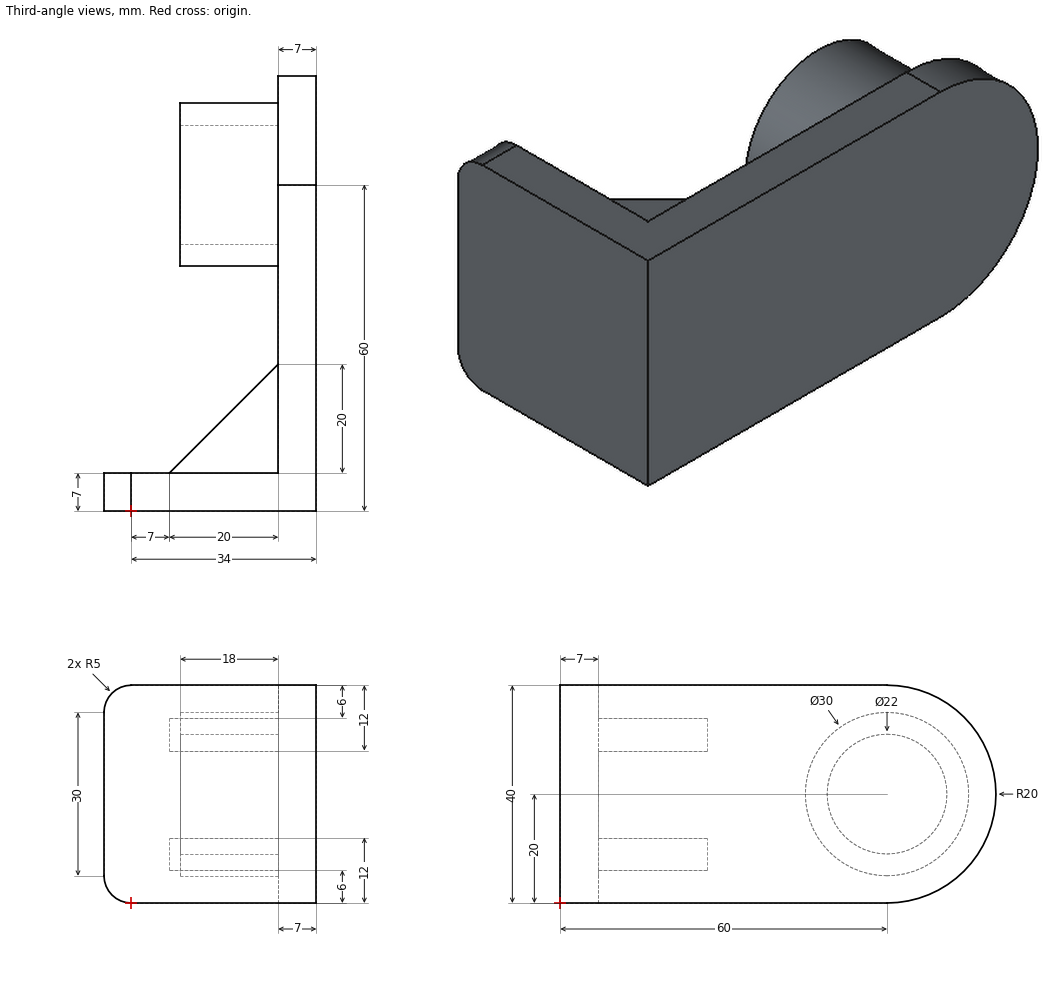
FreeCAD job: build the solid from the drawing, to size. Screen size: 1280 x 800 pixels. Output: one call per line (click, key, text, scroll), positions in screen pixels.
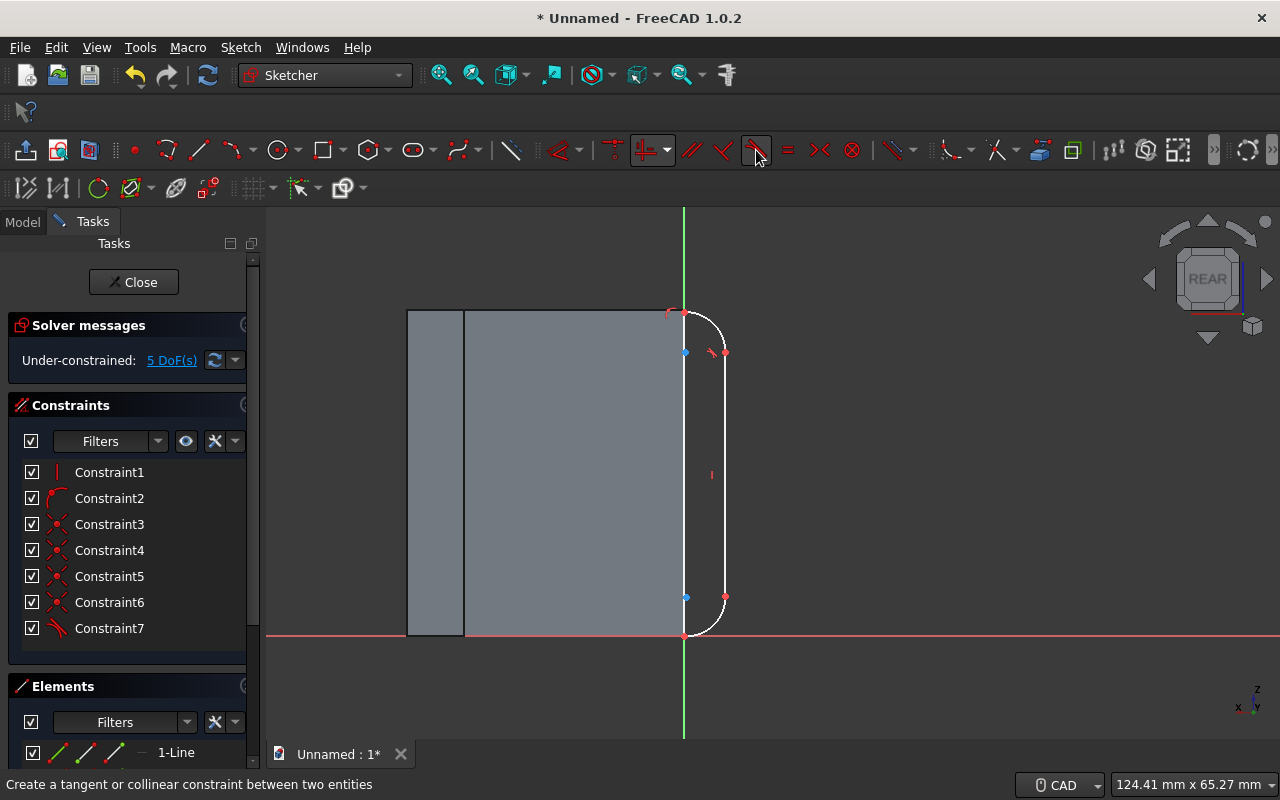
click(725, 523)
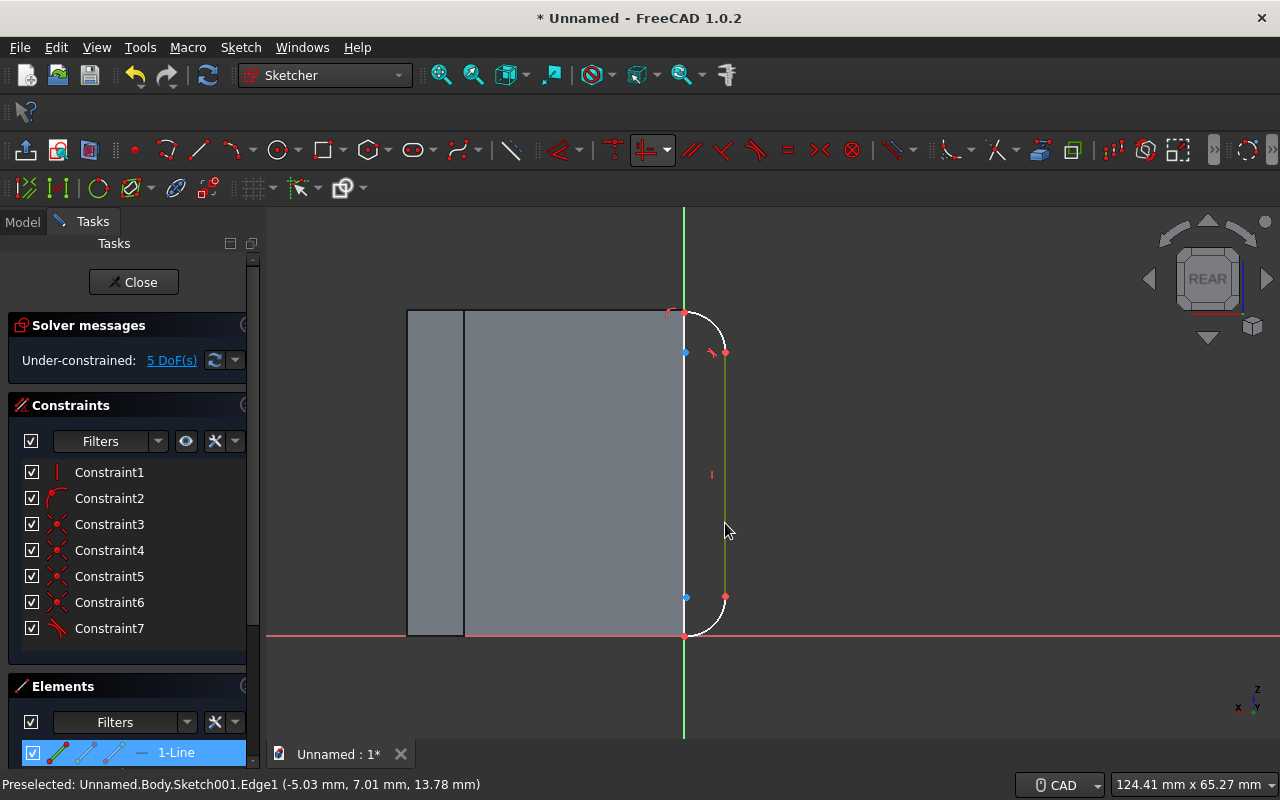
click(703, 633)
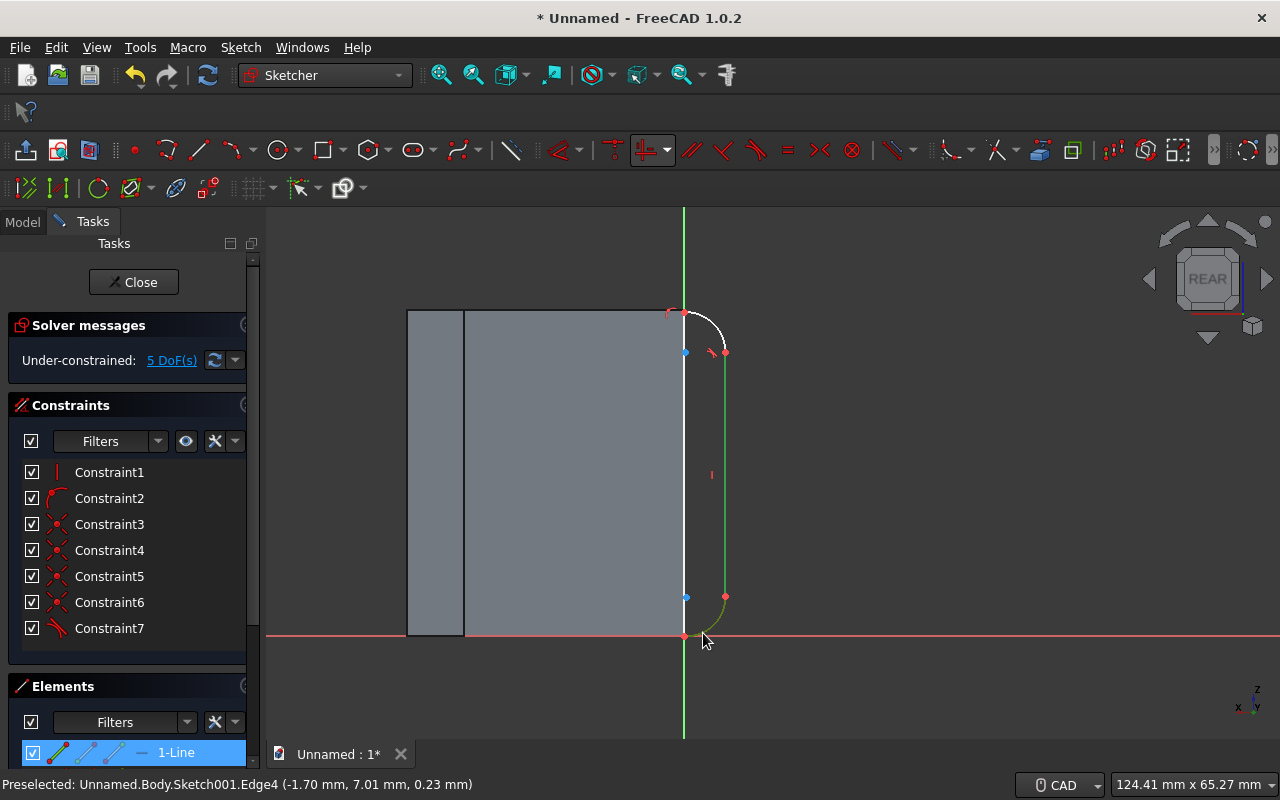
click(756, 150)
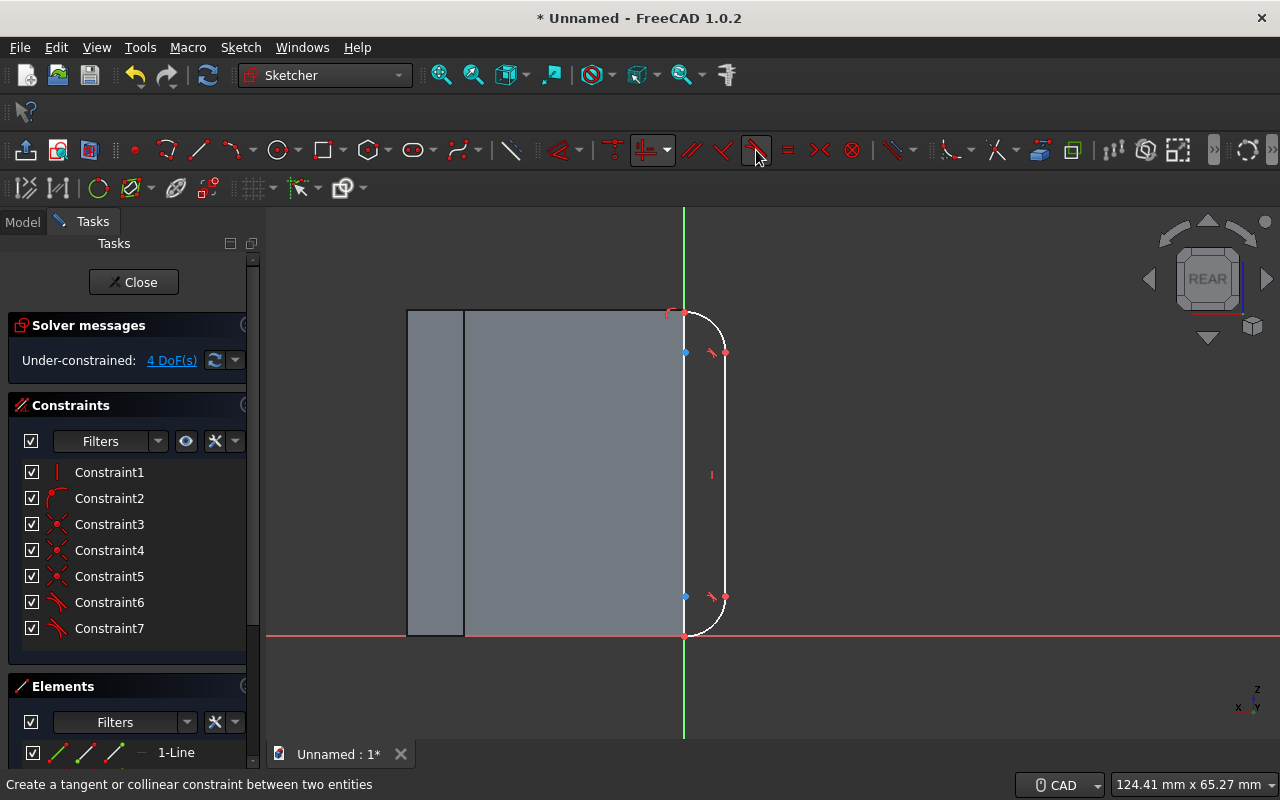
click(721, 334)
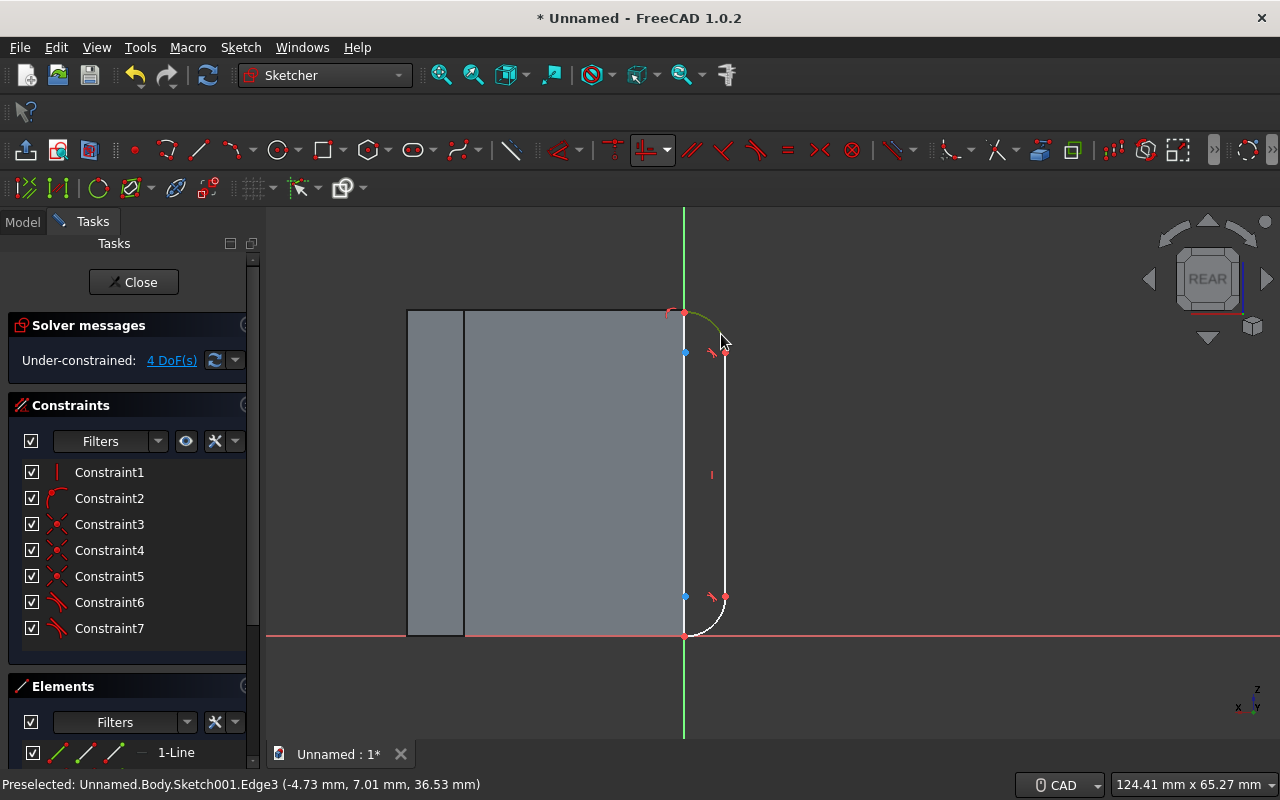
click(703, 632)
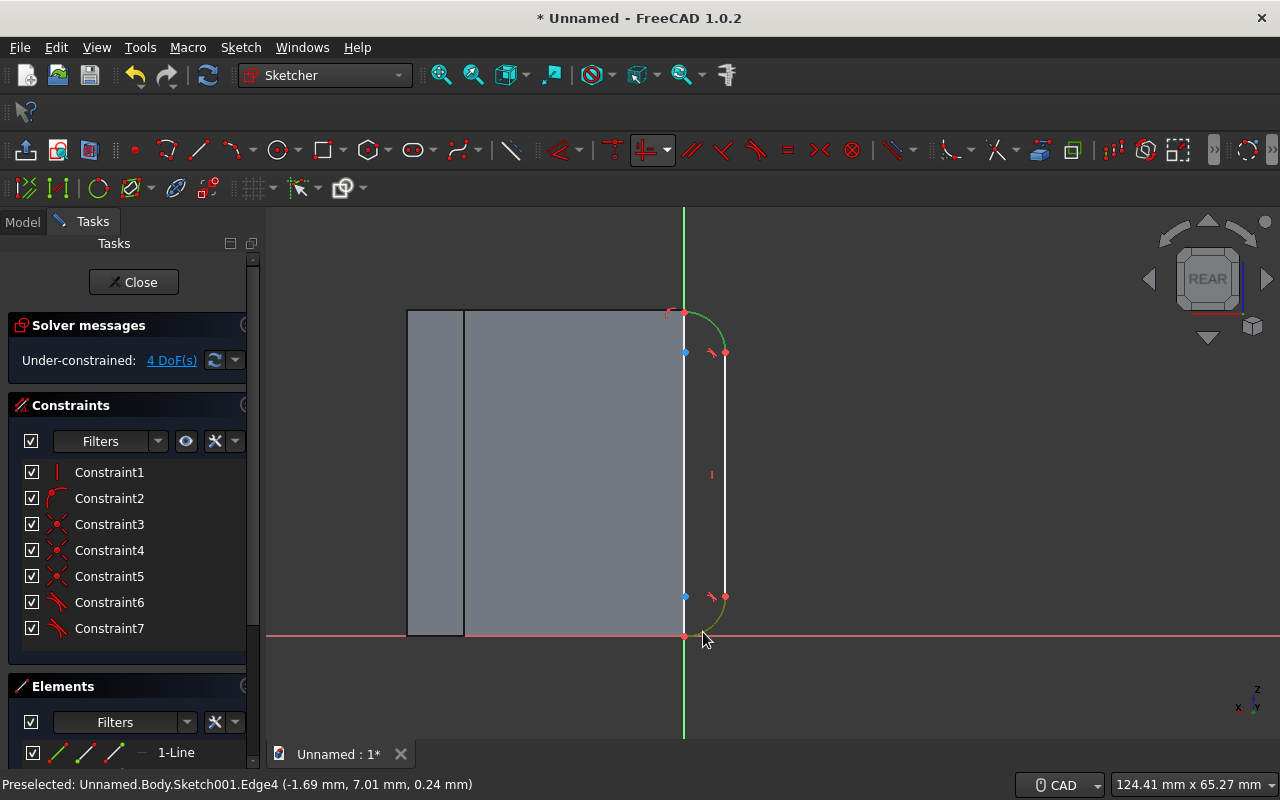
click(788, 150)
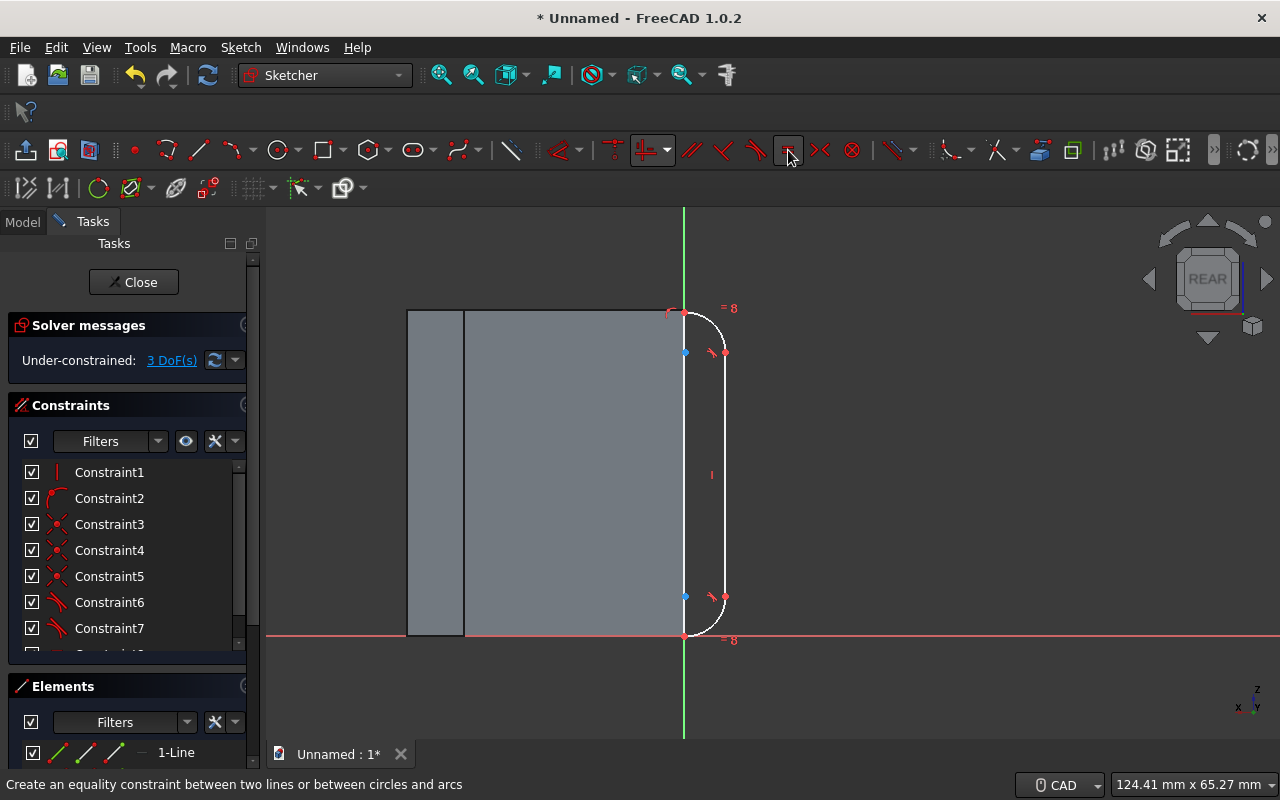
click(686, 352)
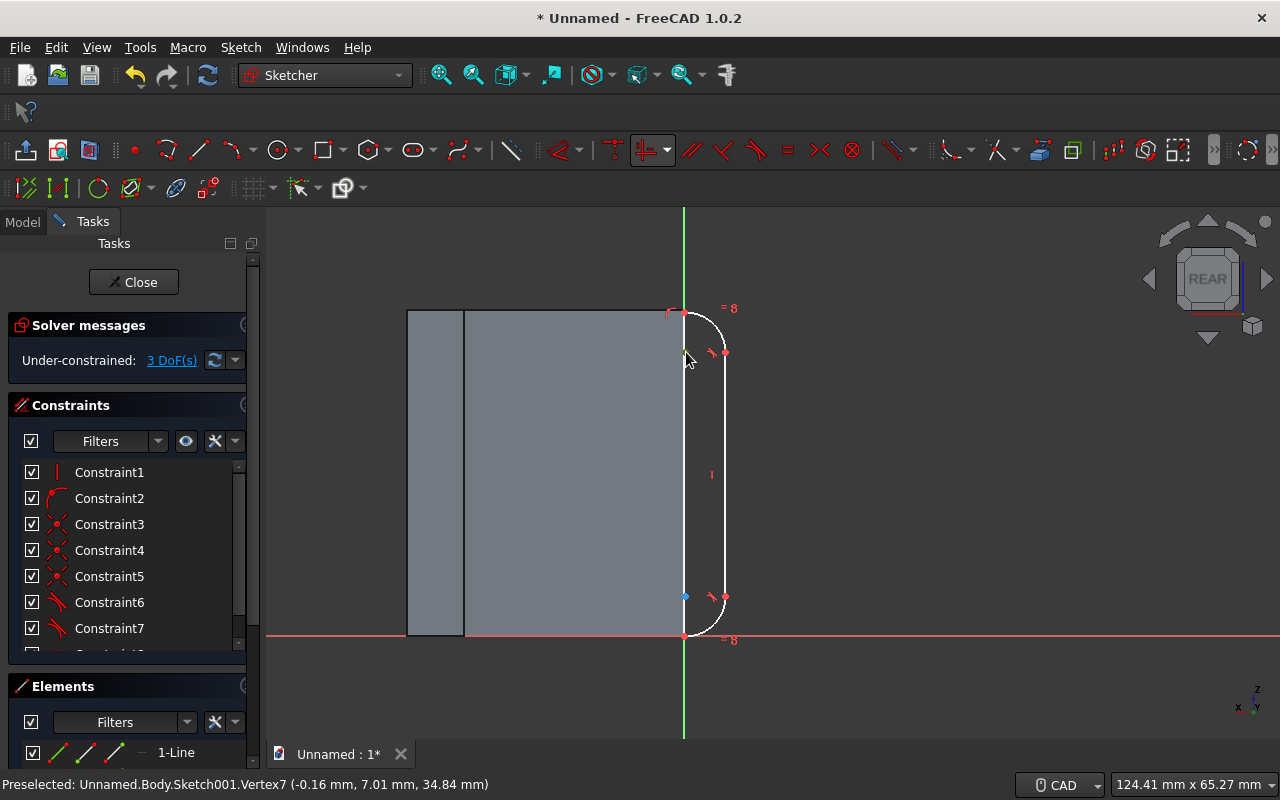
click(684, 677)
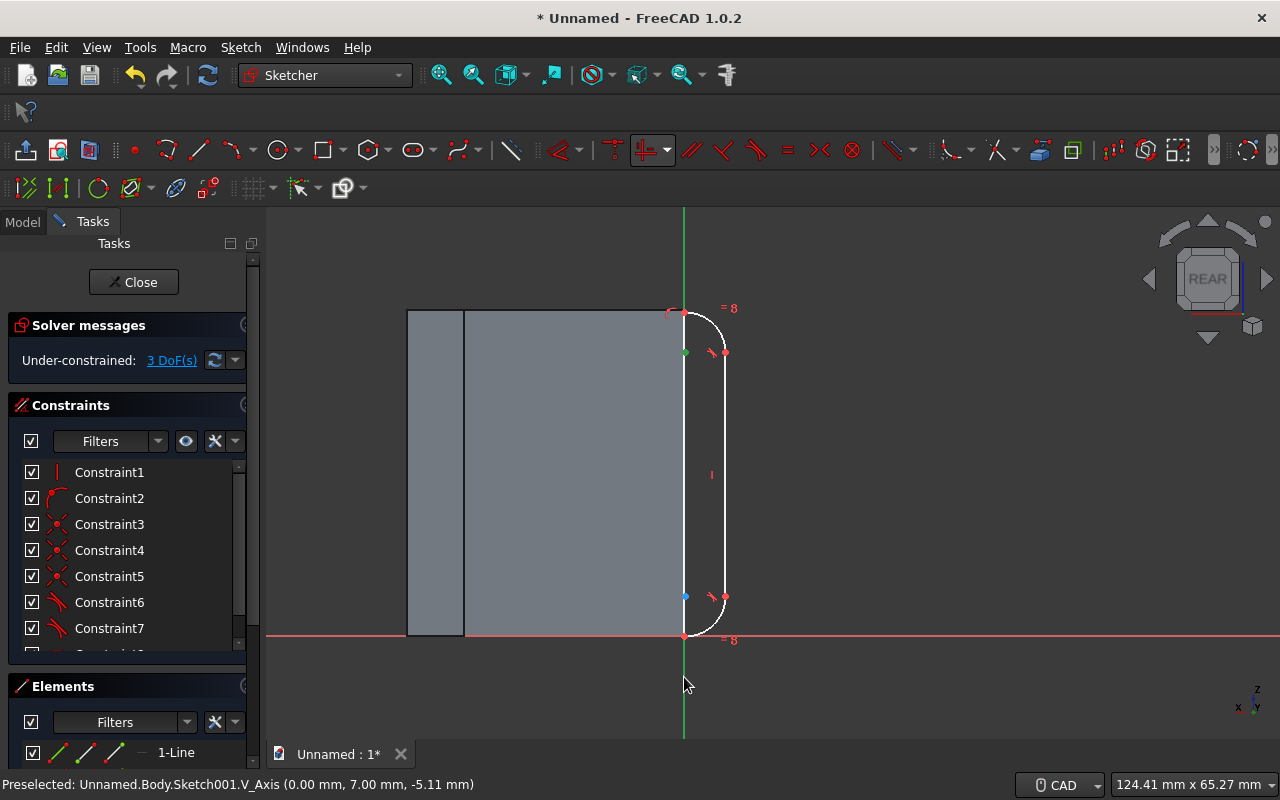
click(614, 150)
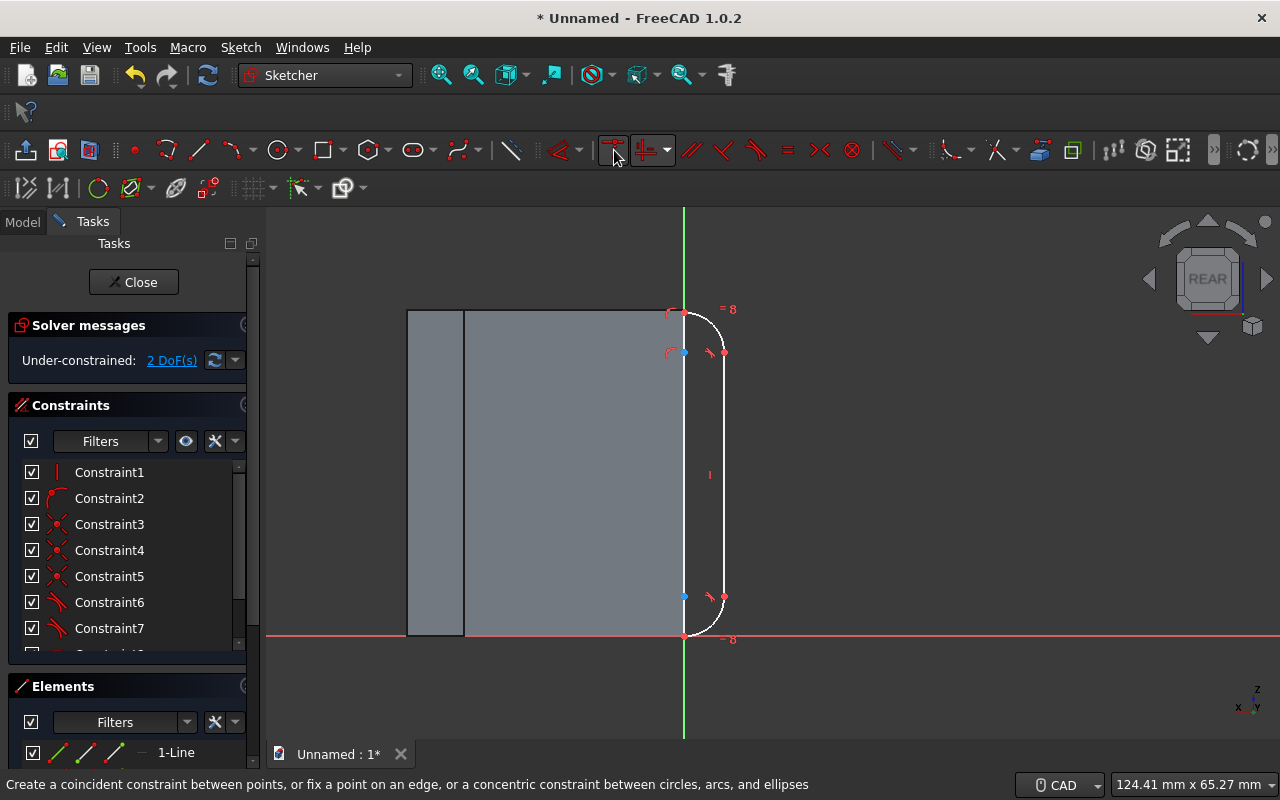
click(558, 150)